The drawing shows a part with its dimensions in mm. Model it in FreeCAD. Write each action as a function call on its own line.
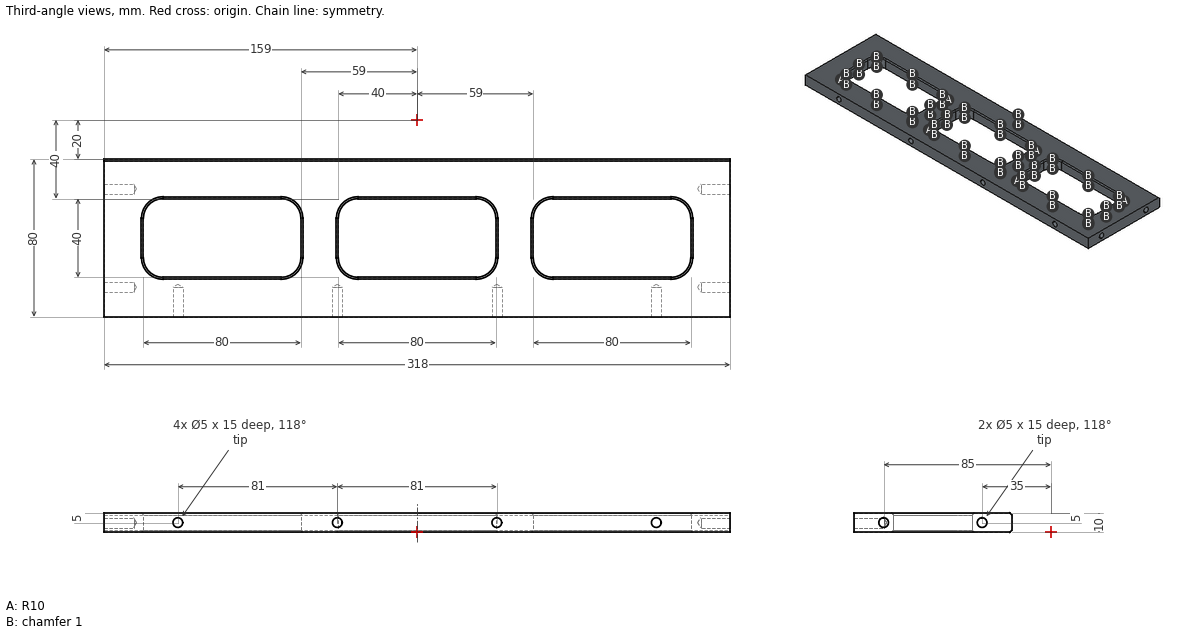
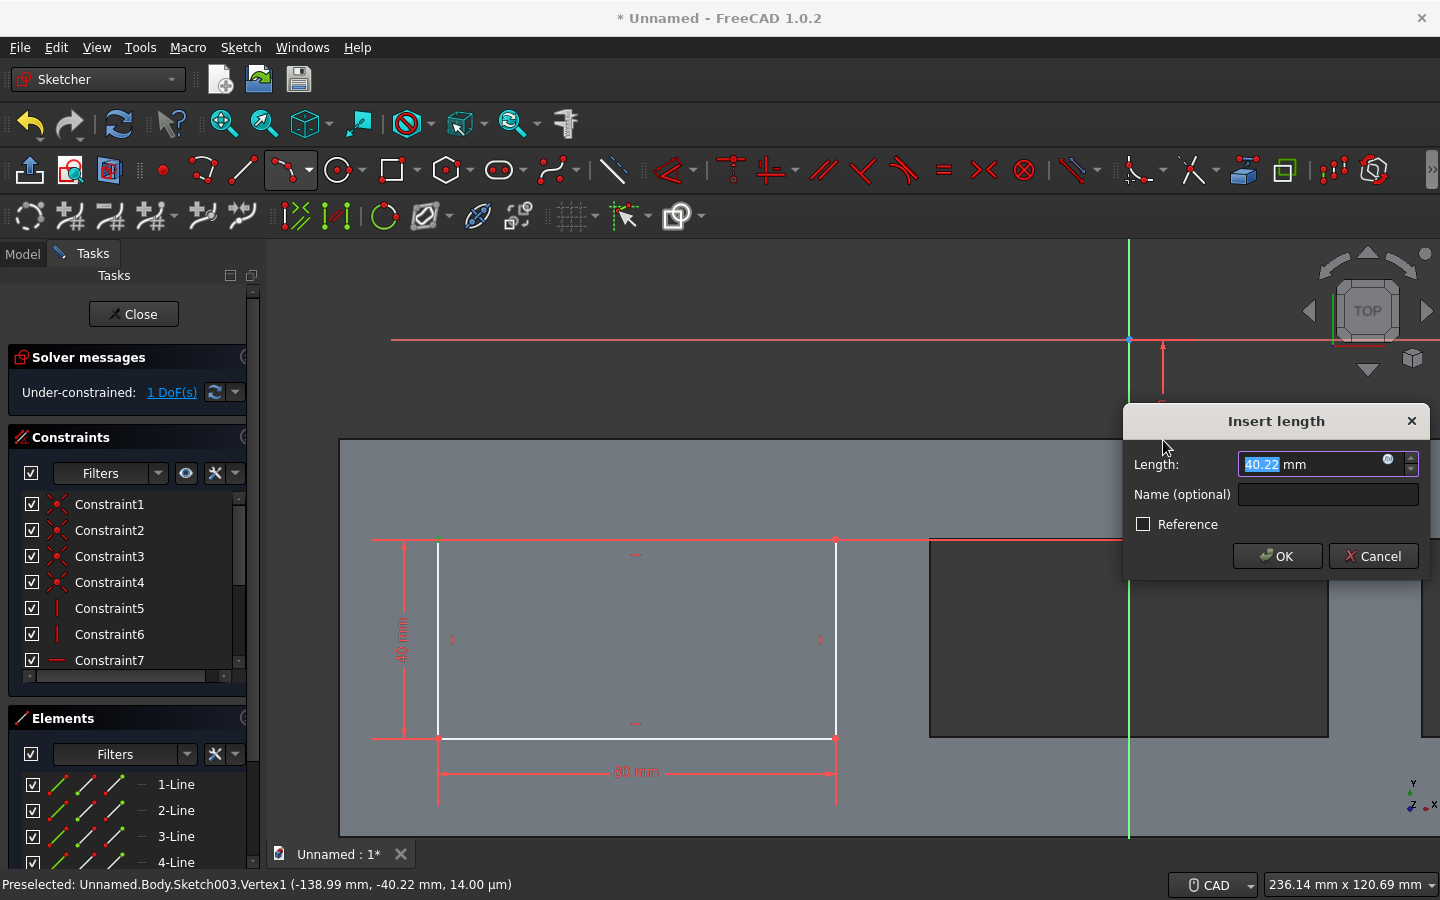
text(40)
key(Return)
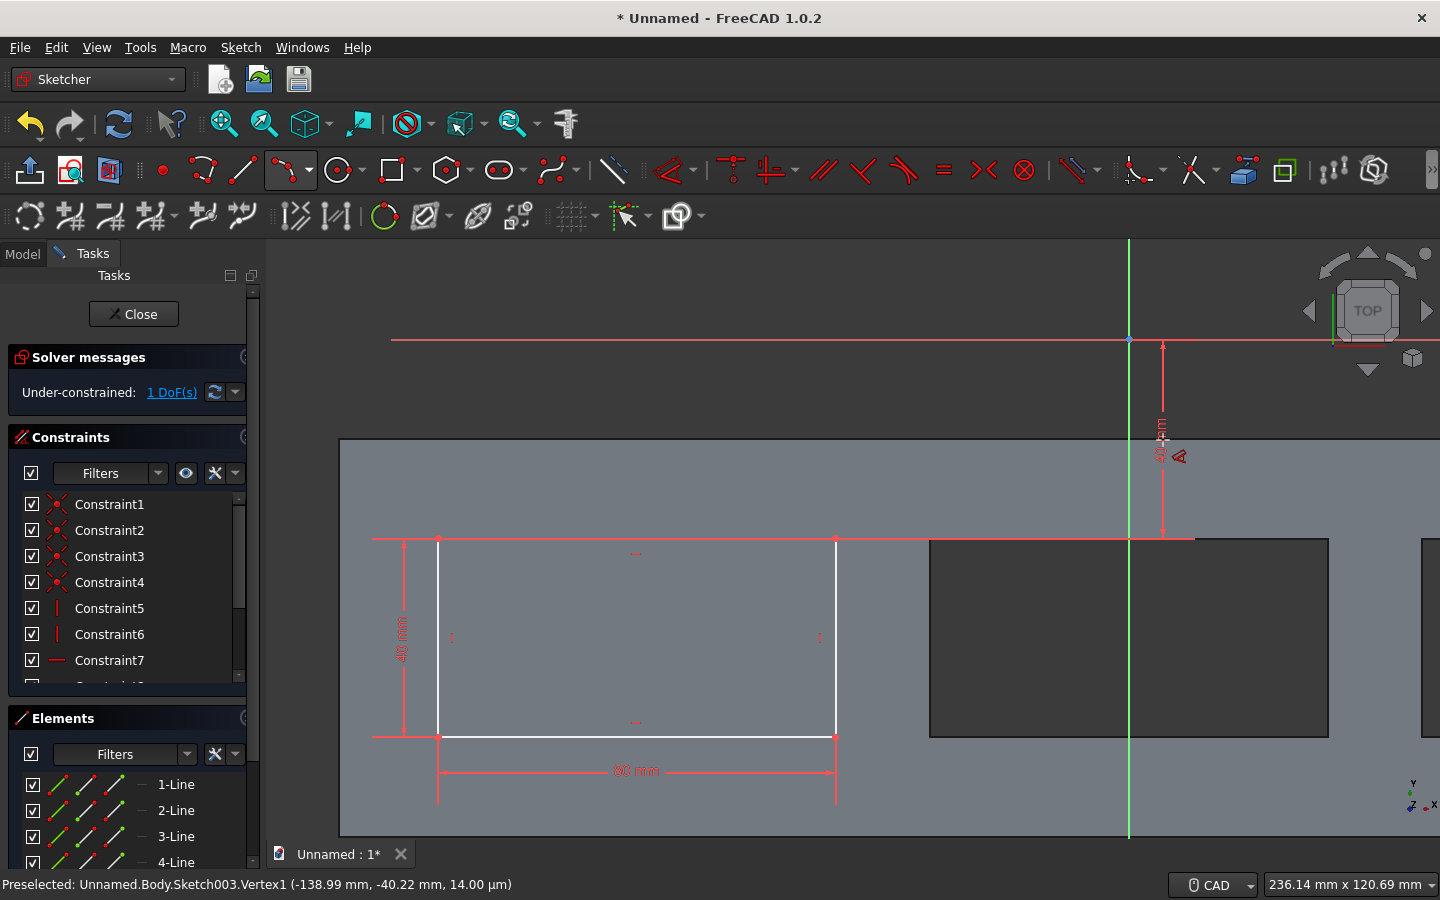
click(836, 737)
click(982, 306)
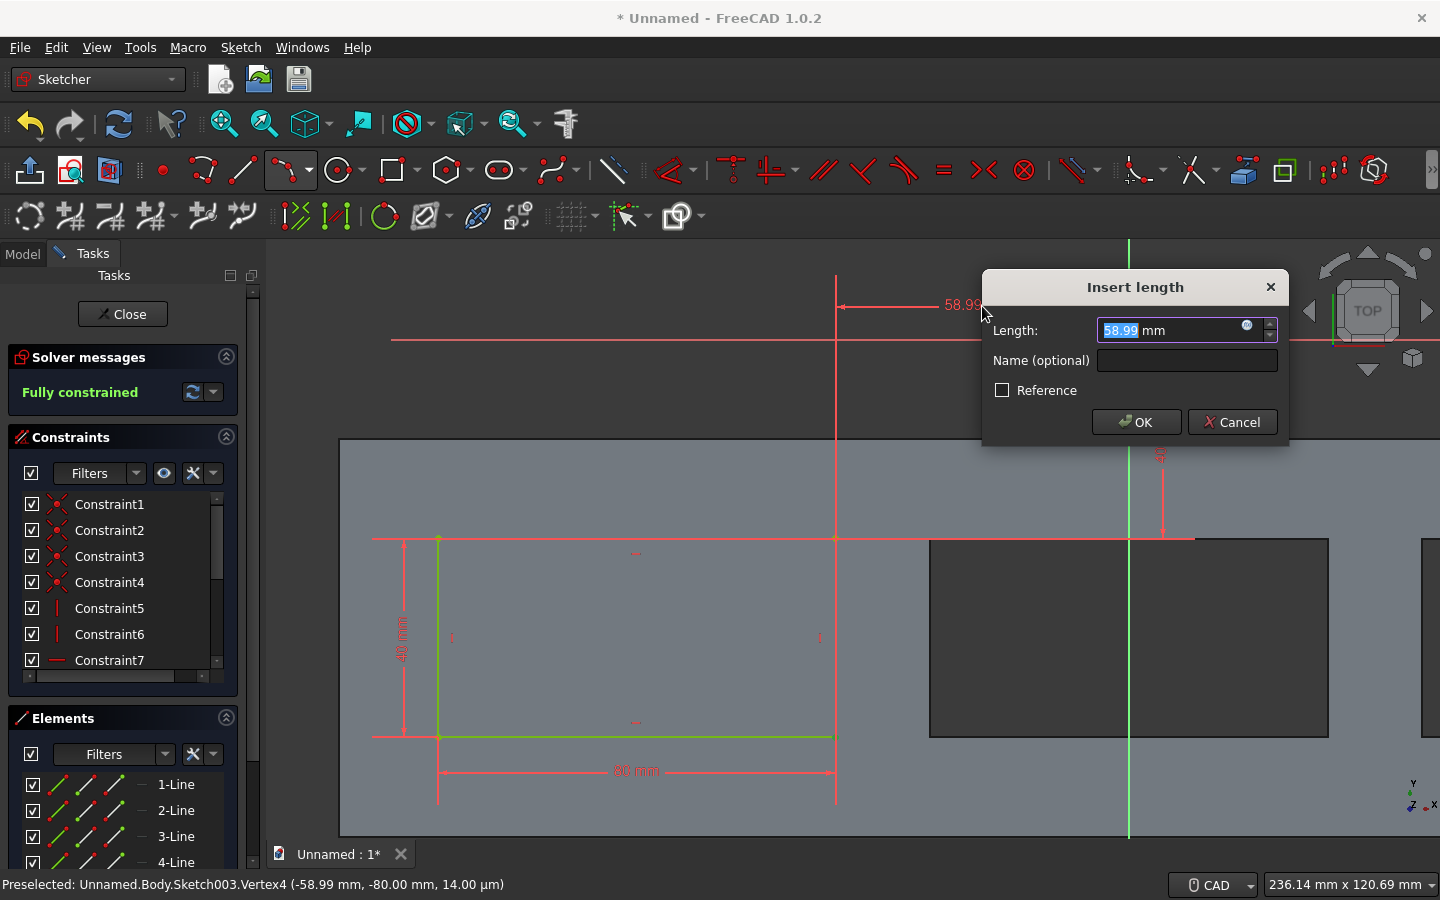
text(59)
key(Return)
key(Escape)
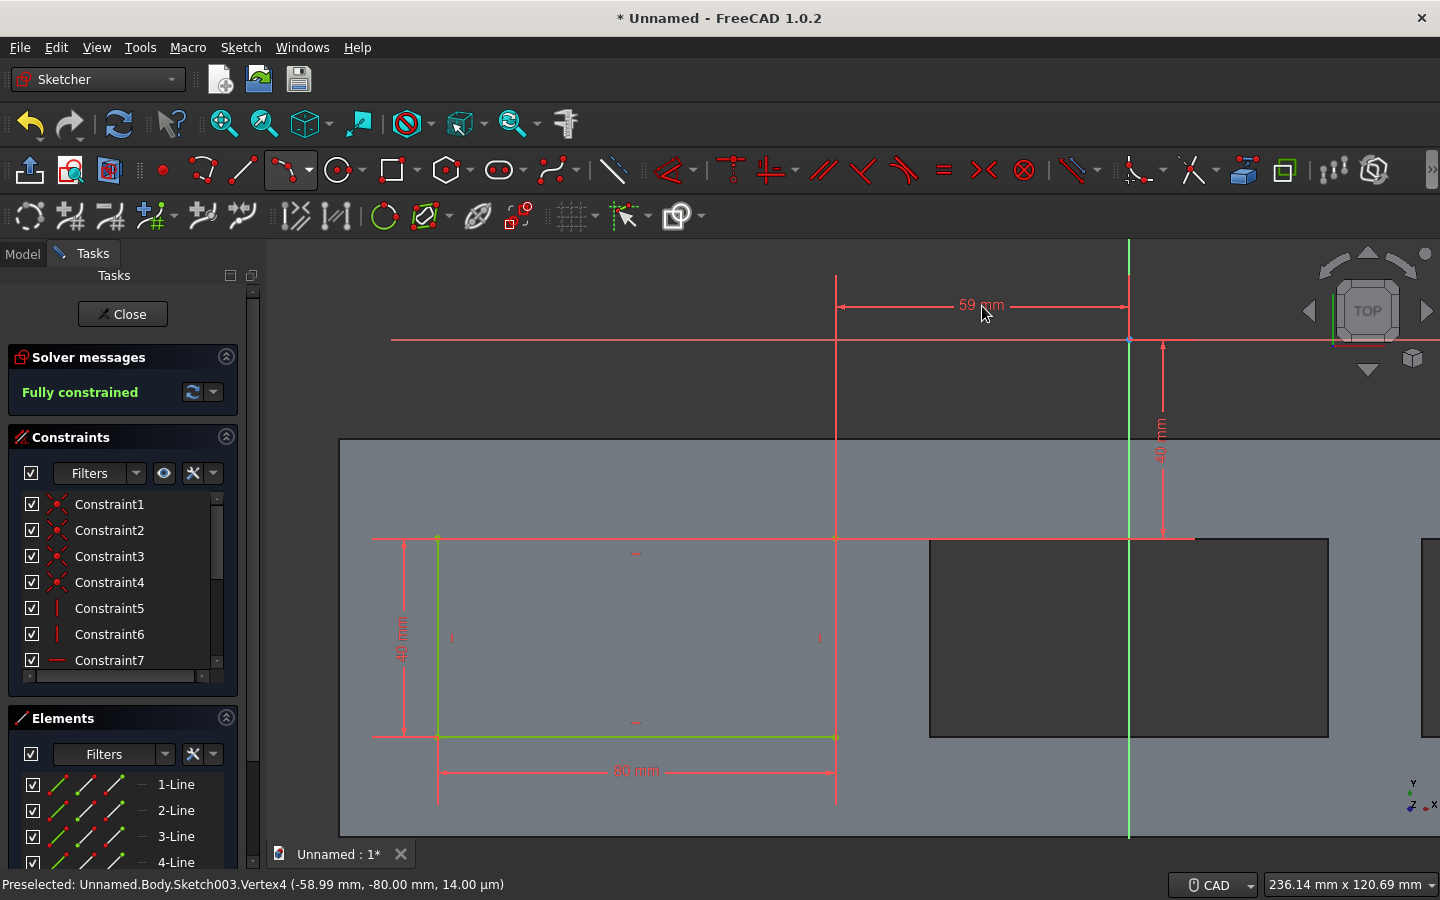
click(123, 314)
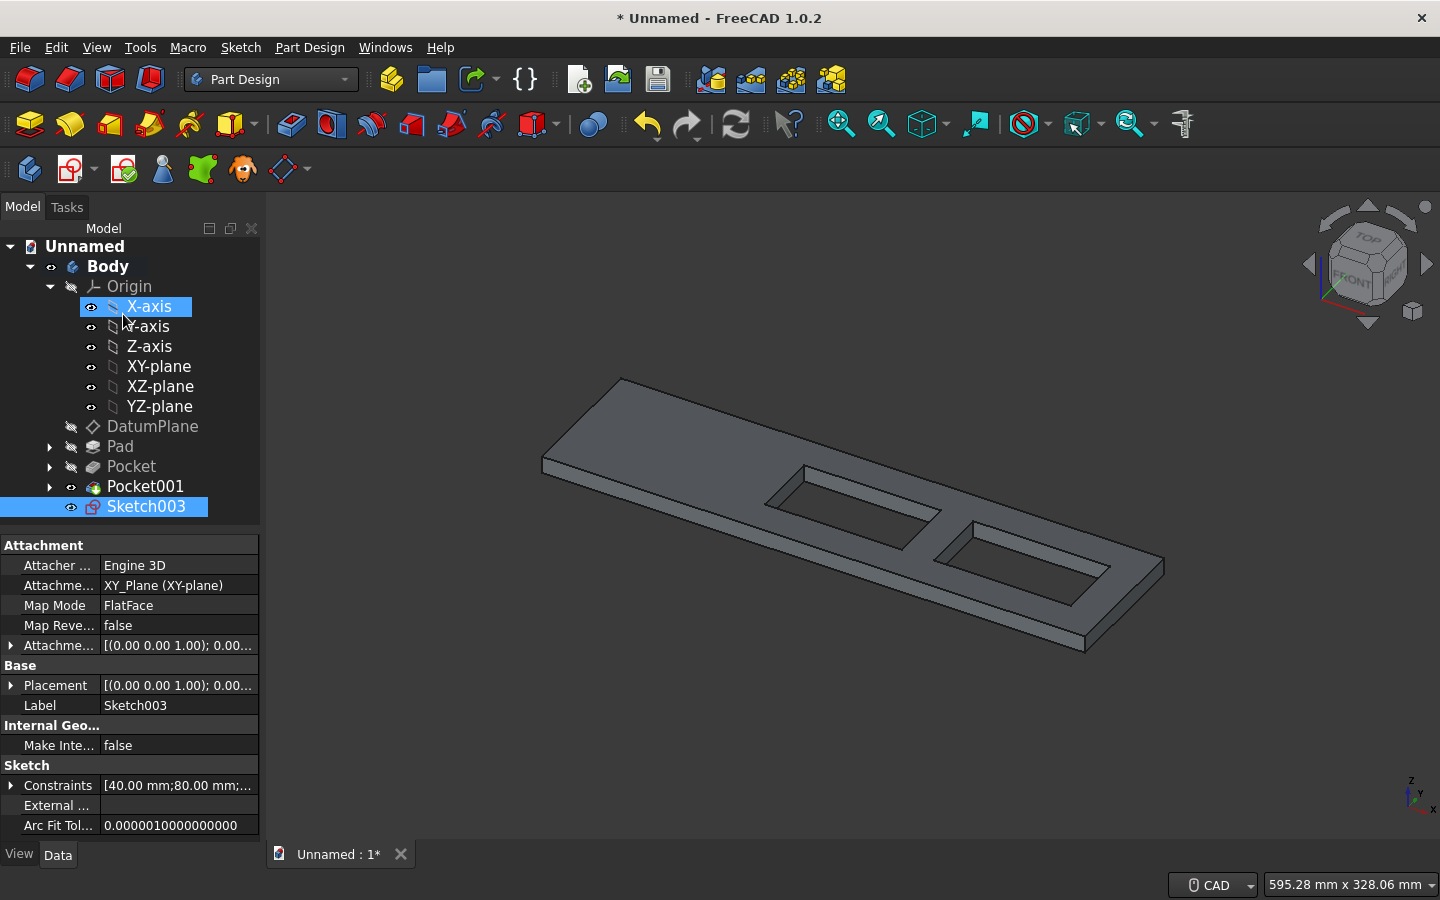
click(292, 124)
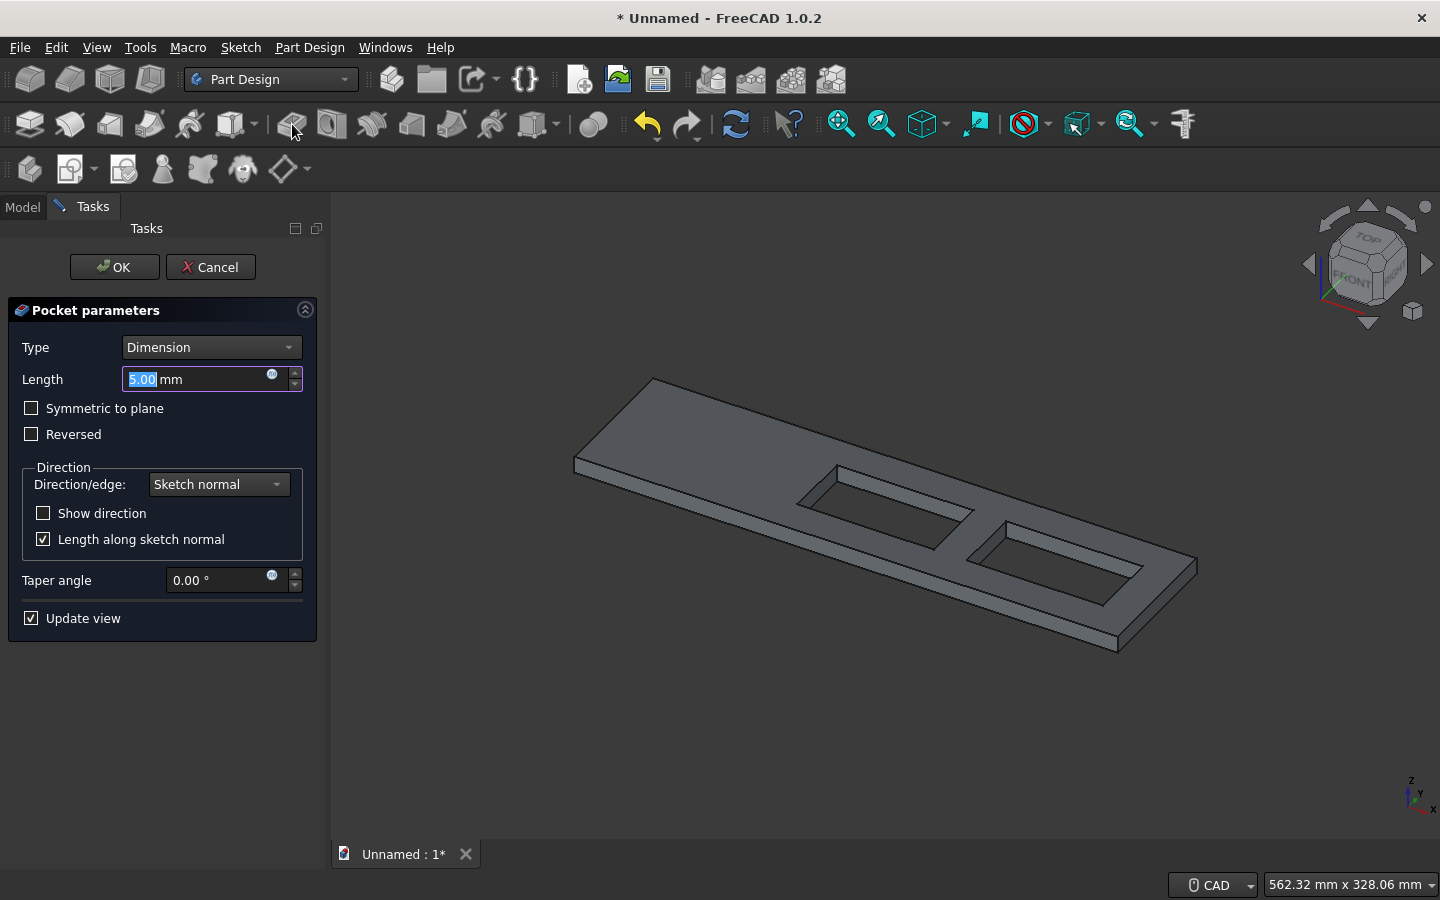
click(212, 348)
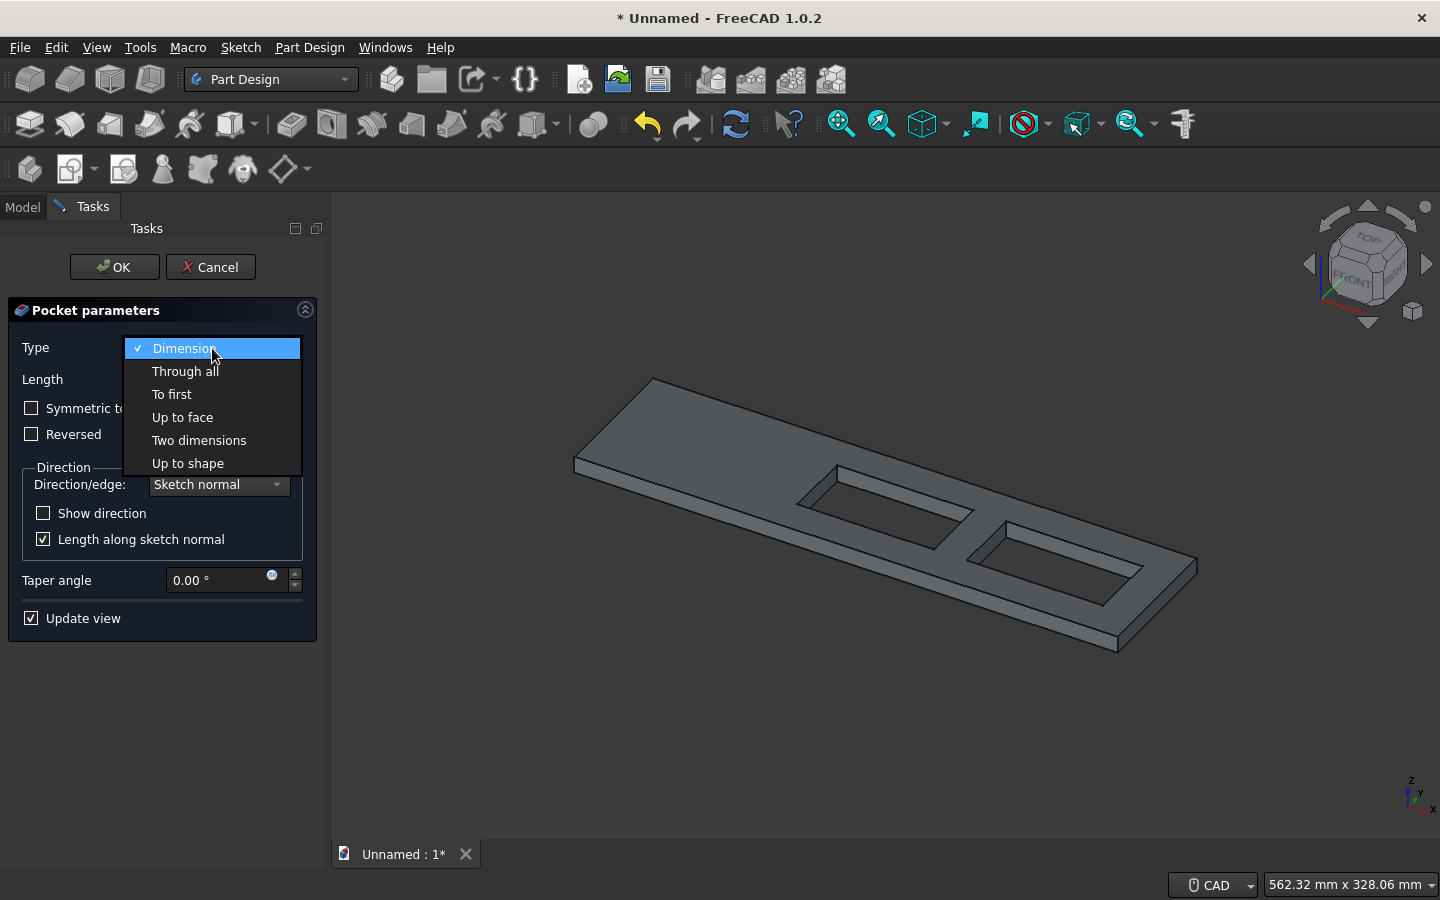
click(212, 372)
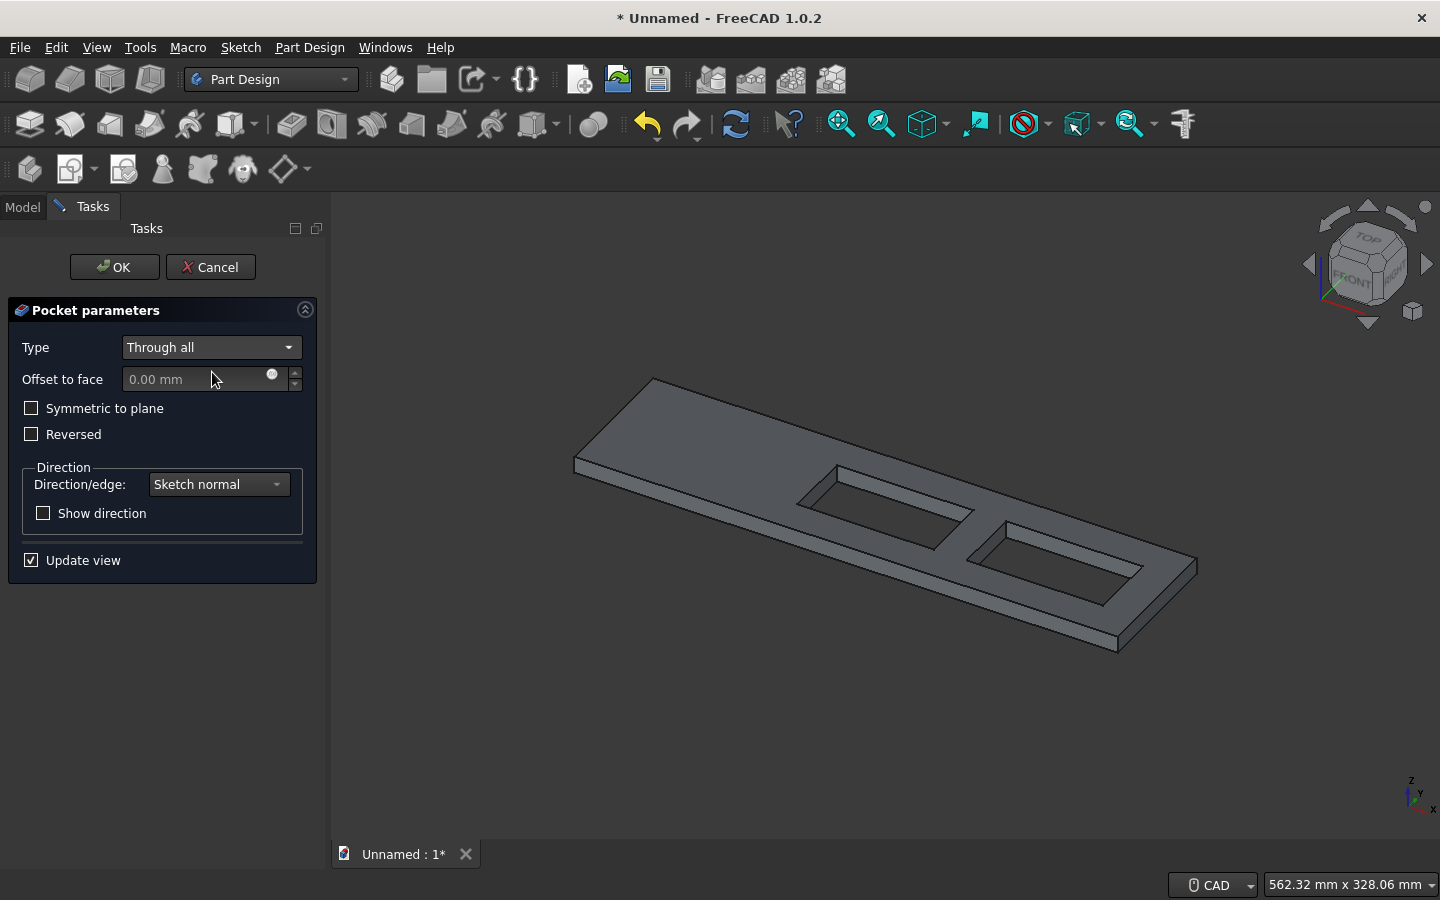
click(30, 434)